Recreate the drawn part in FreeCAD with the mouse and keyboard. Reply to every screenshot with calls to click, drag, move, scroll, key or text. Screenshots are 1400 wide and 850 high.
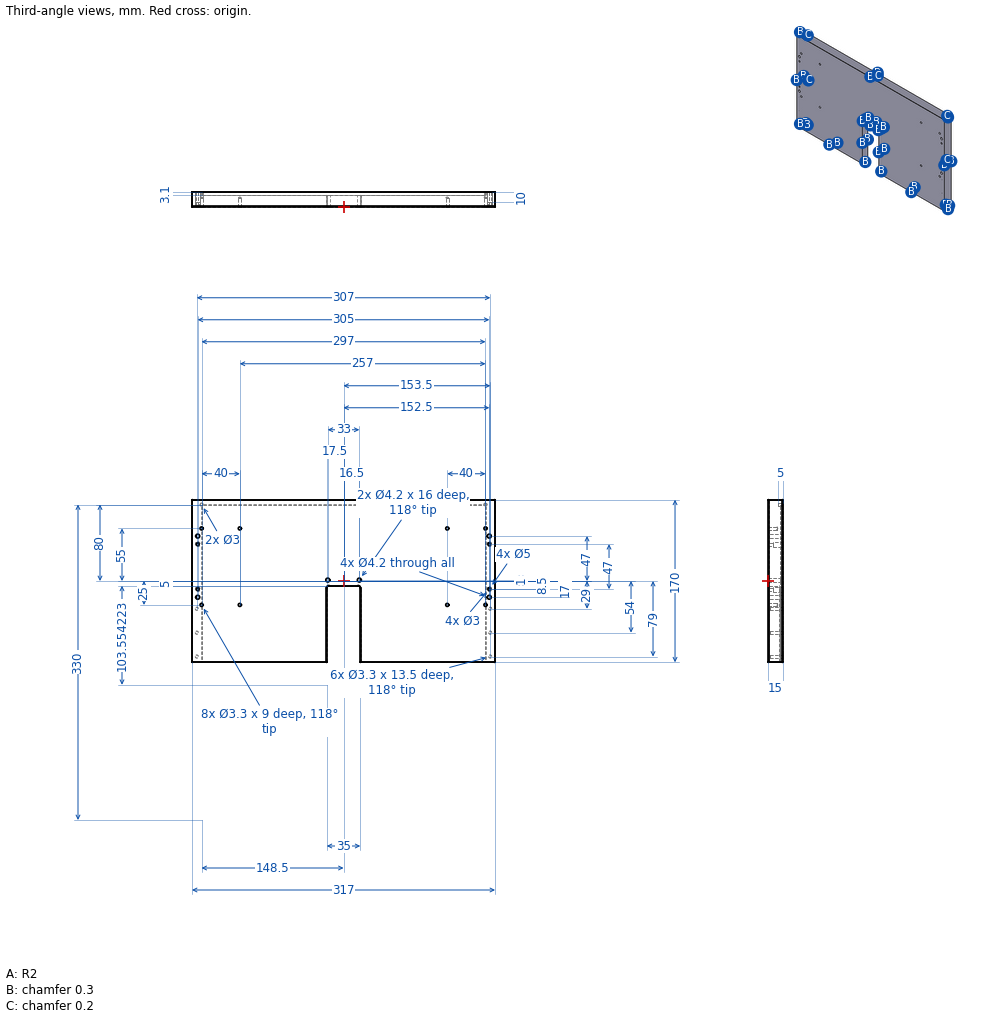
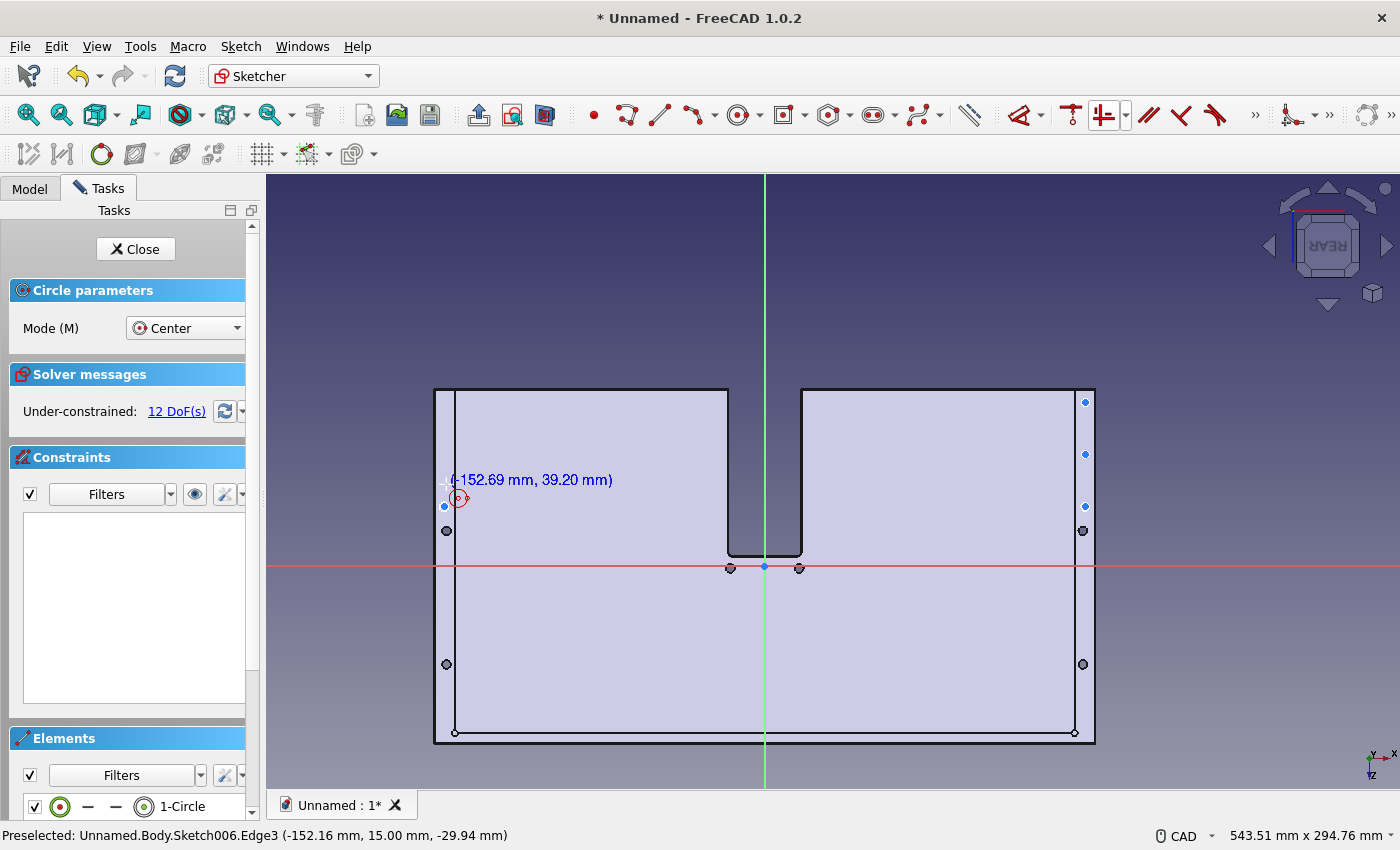
click(444, 454)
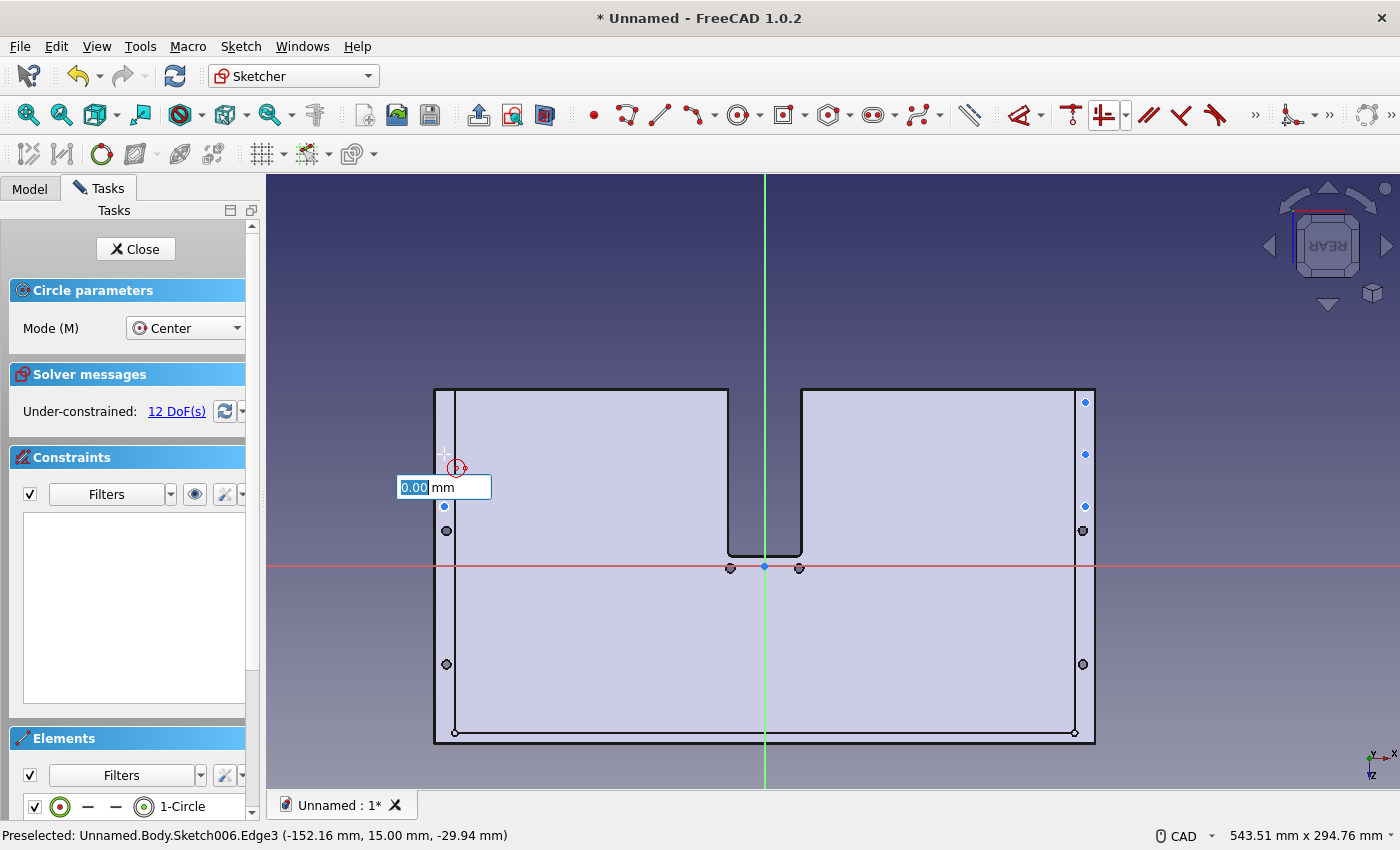
scroll(447, 451, up, 8)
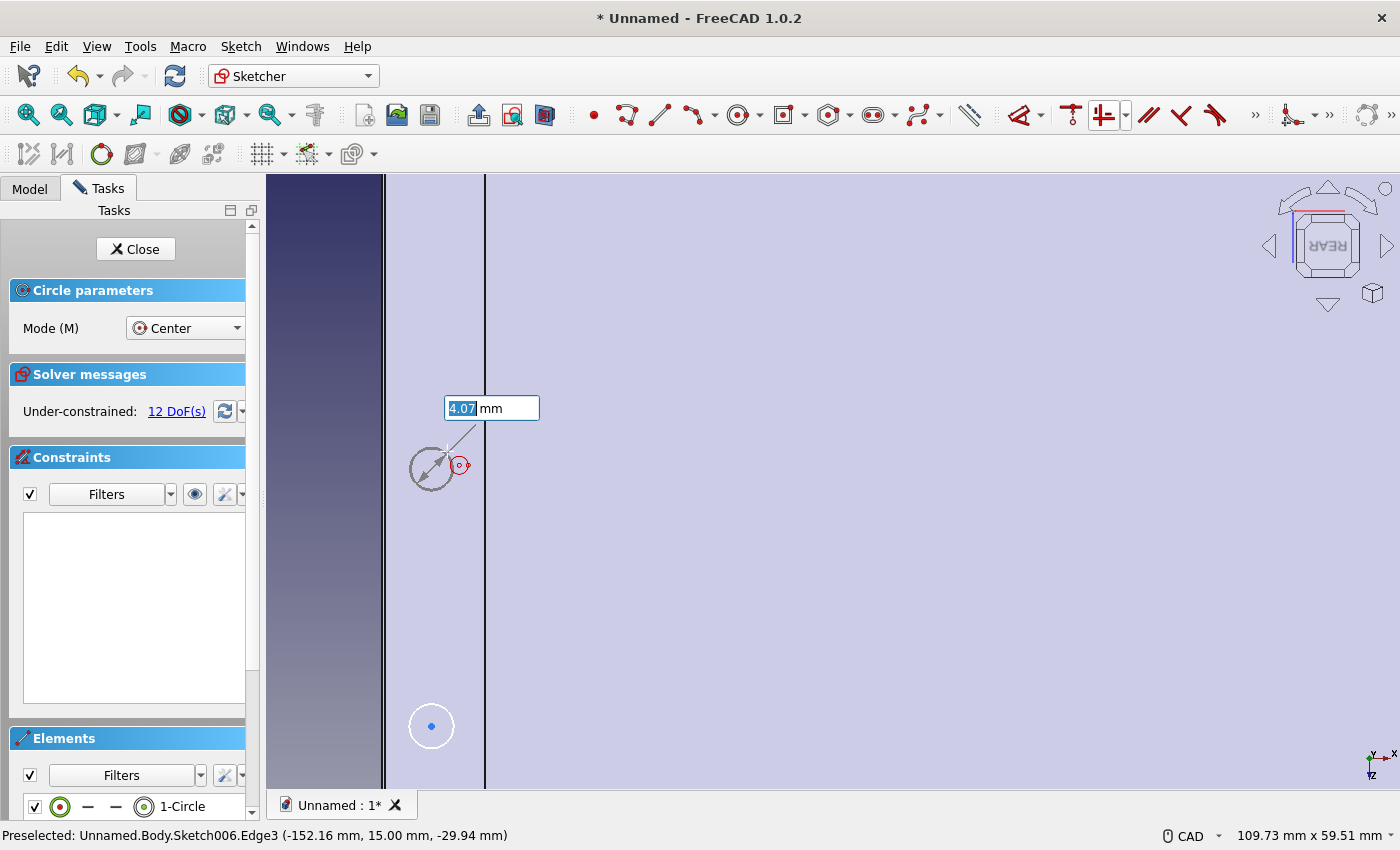
click(446, 451)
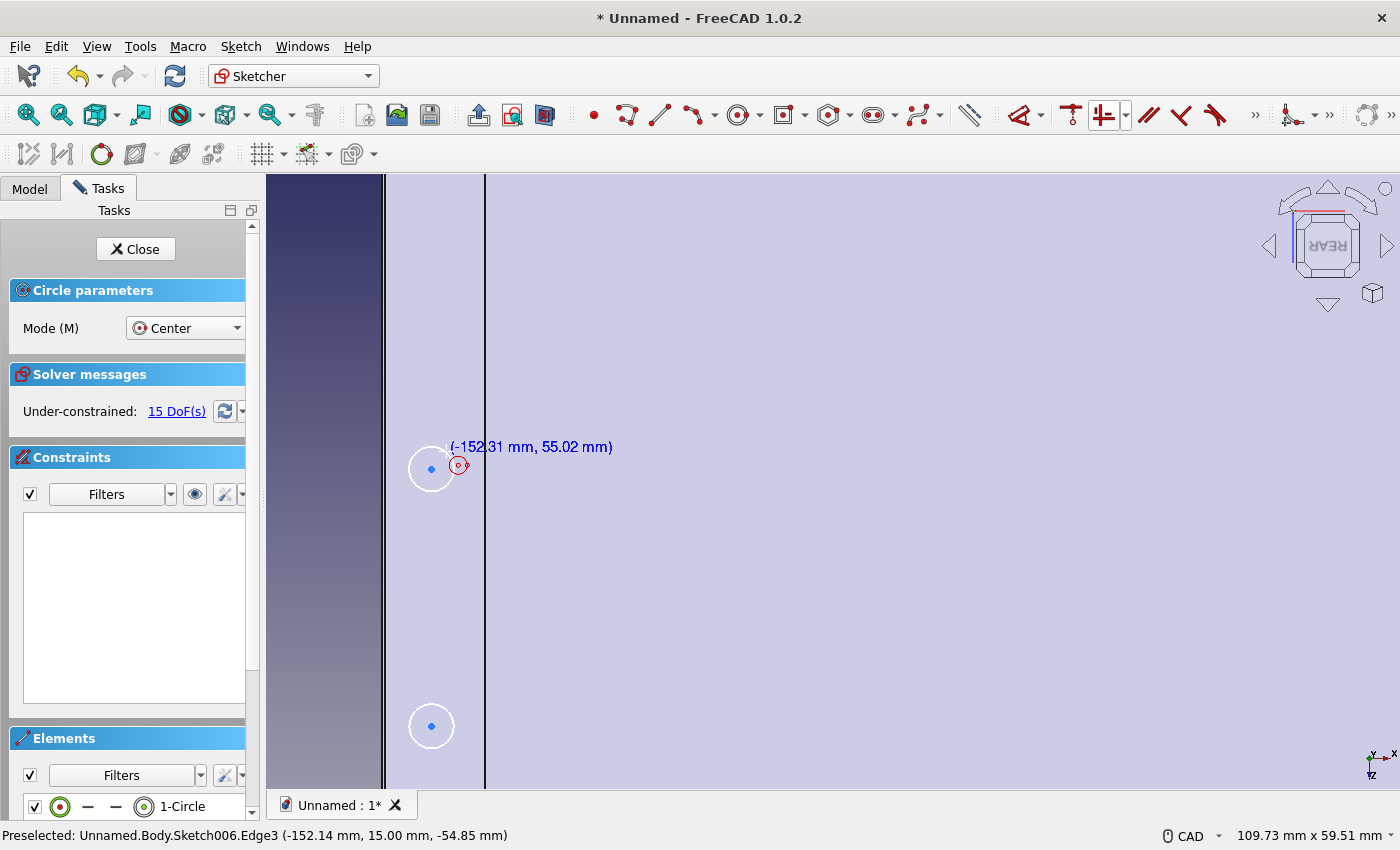
scroll(434, 204, up, 2)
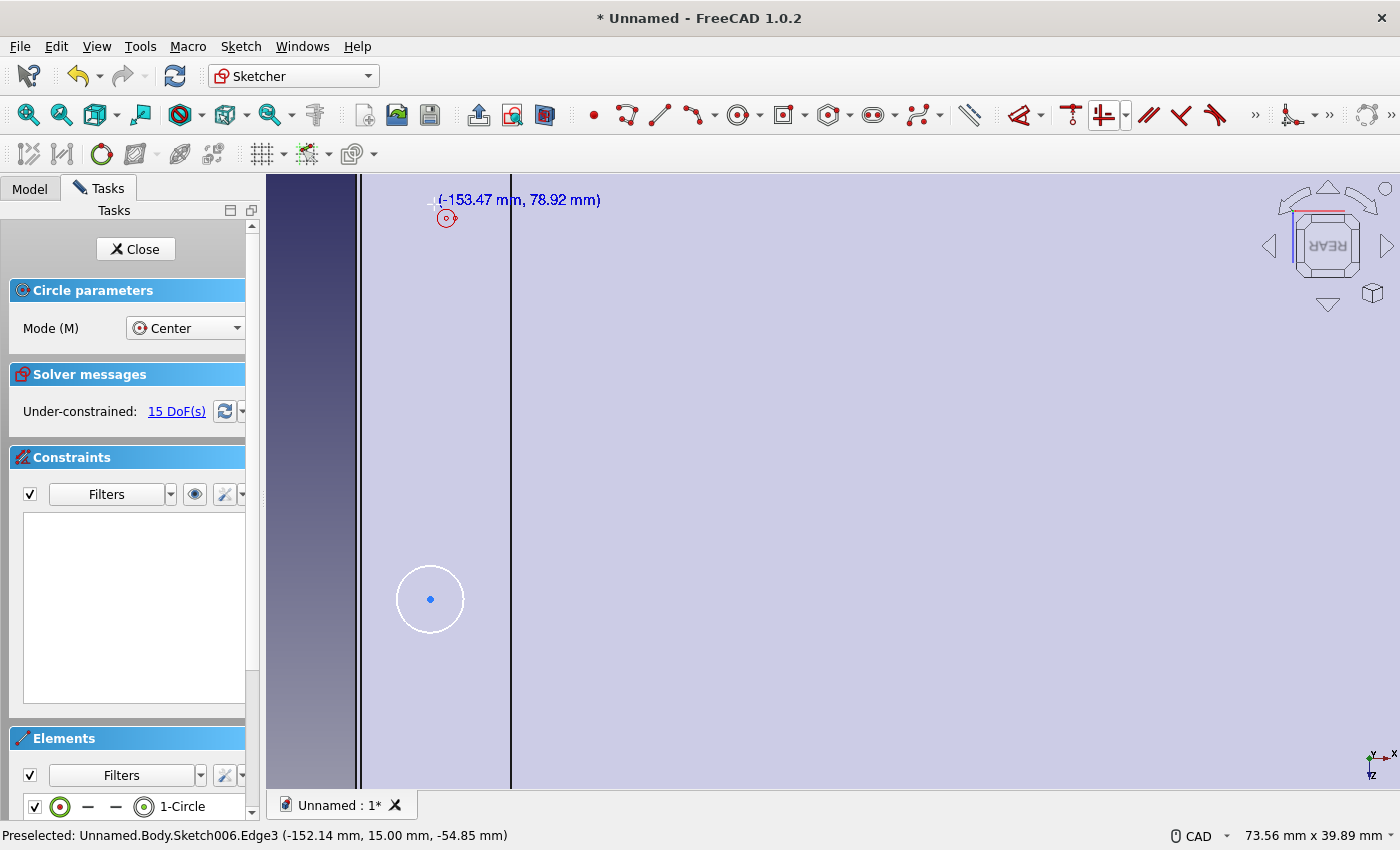
scroll(446, 432, down, 10)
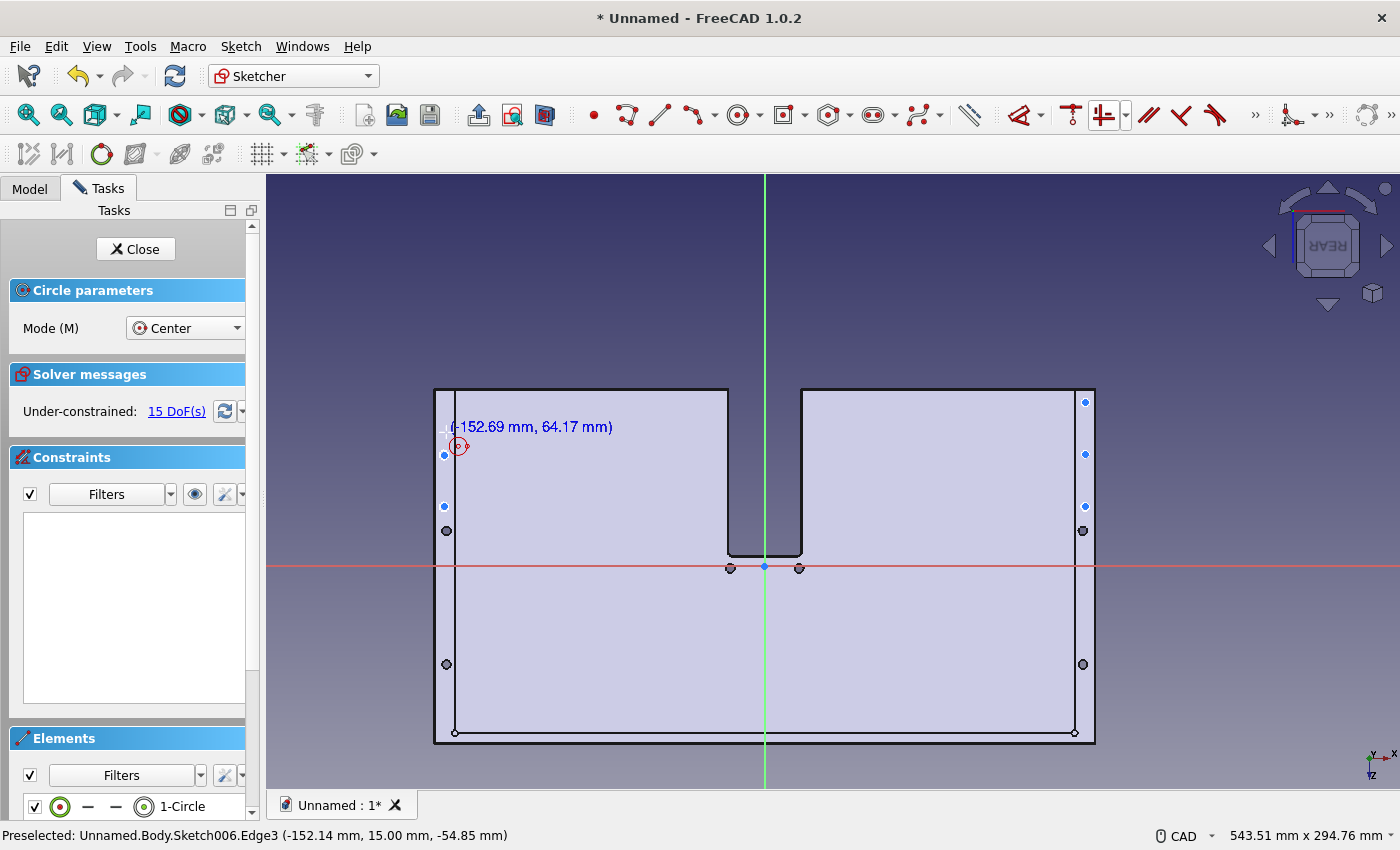
click(444, 402)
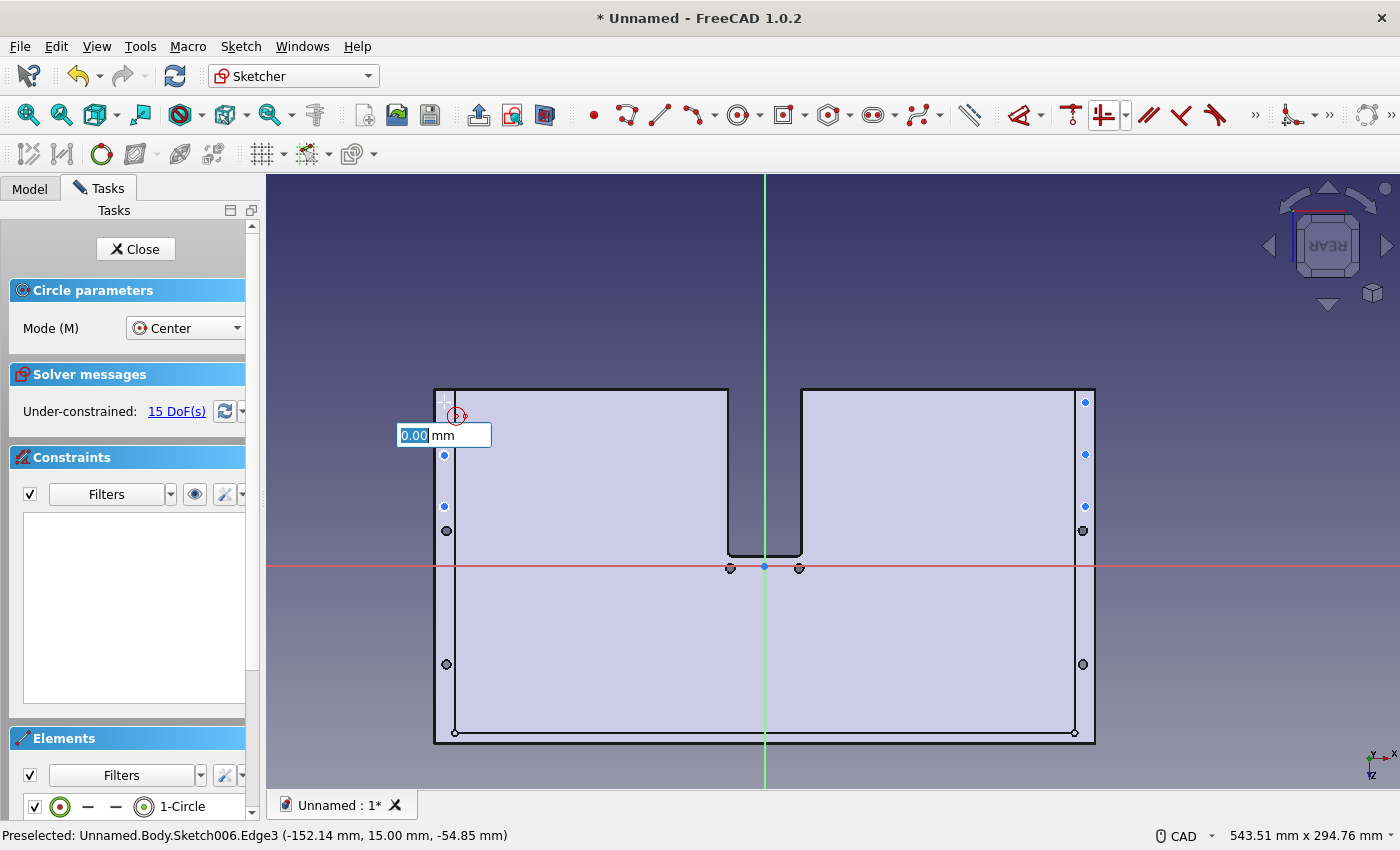
scroll(447, 399, up, 8)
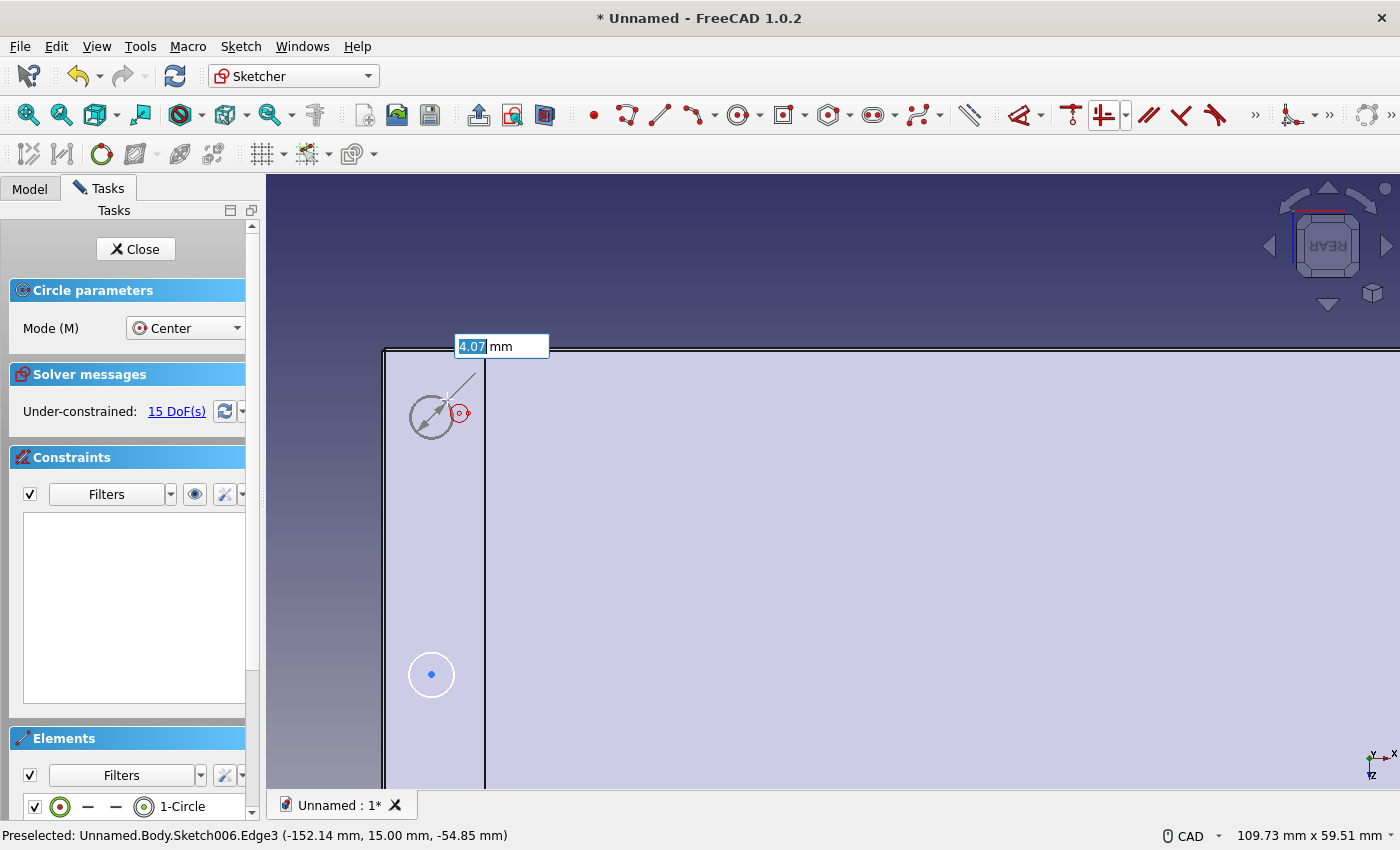
click(446, 398)
key(Escape)